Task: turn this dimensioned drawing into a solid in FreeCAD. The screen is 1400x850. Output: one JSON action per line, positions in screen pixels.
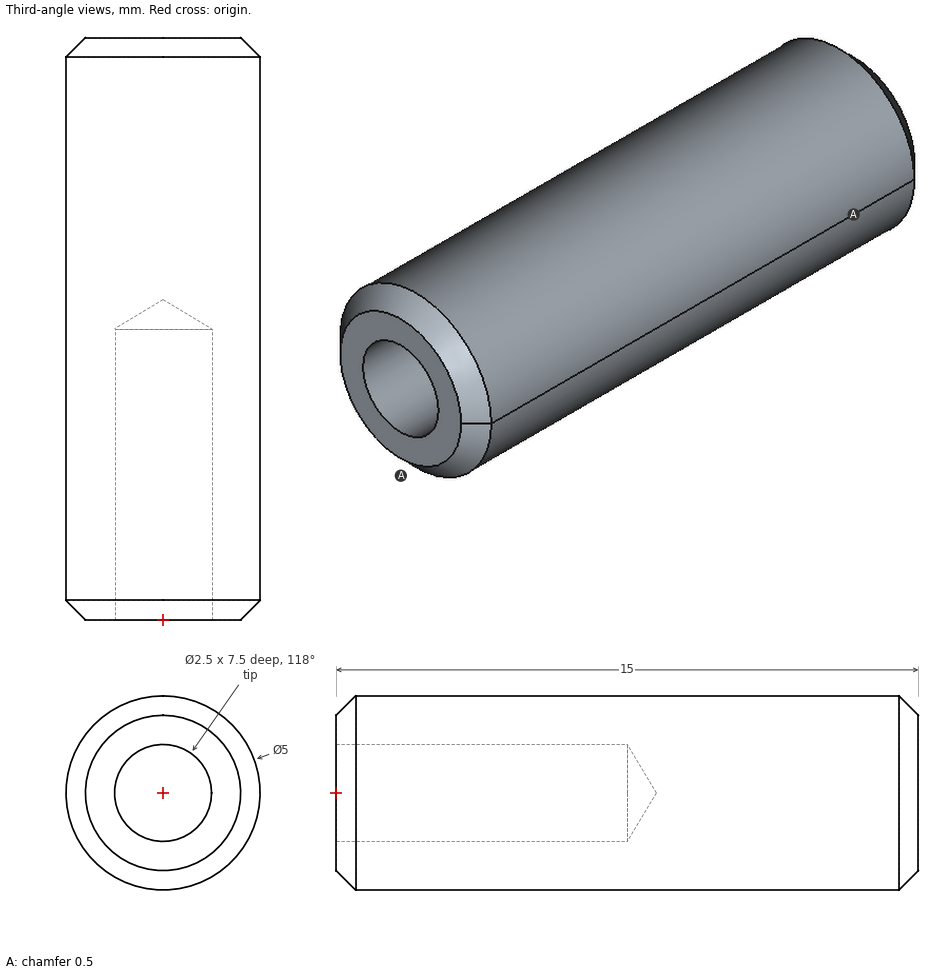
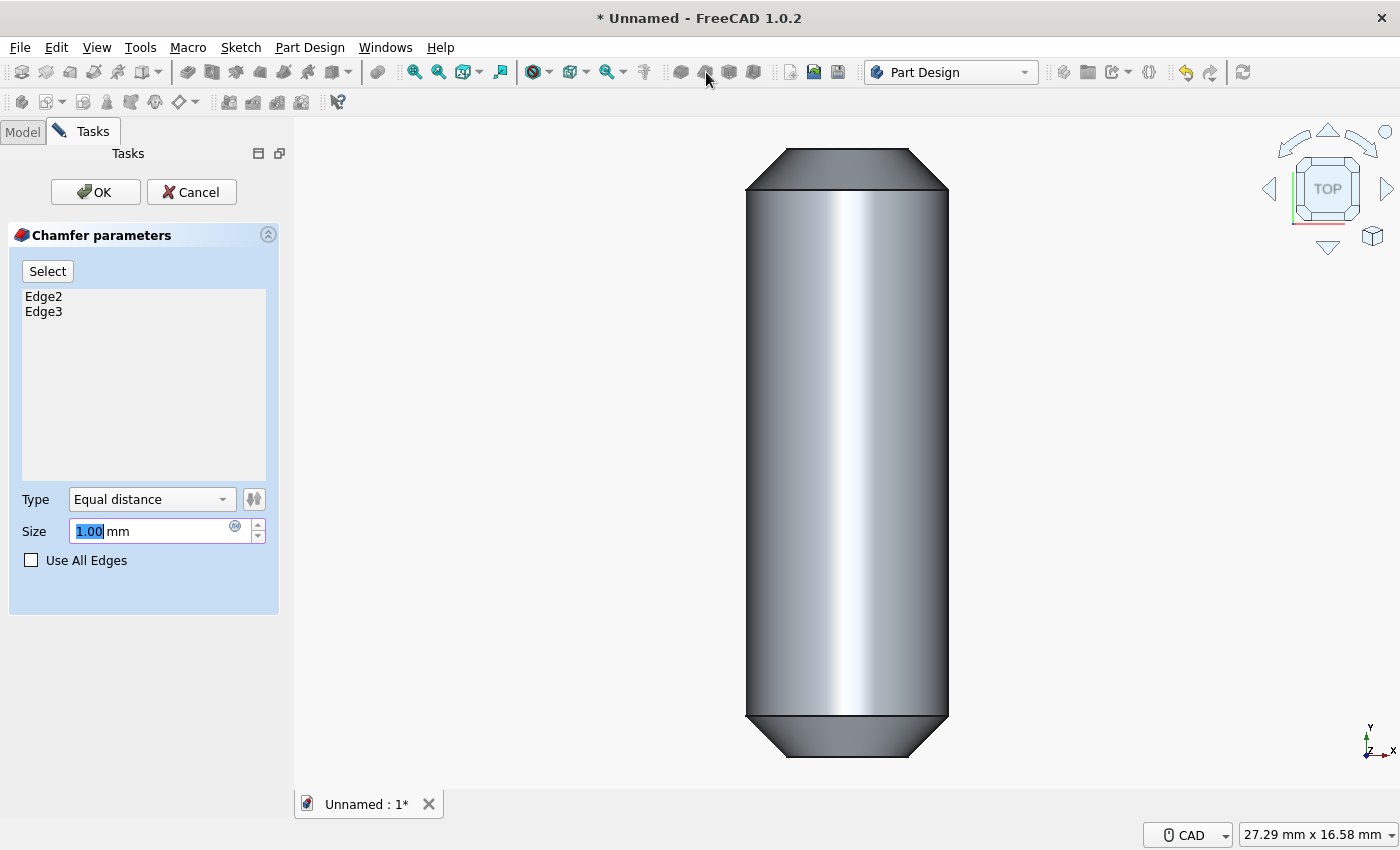
{"action": "type", "text": "0.5"}
{"action": "key", "text": "Tab"}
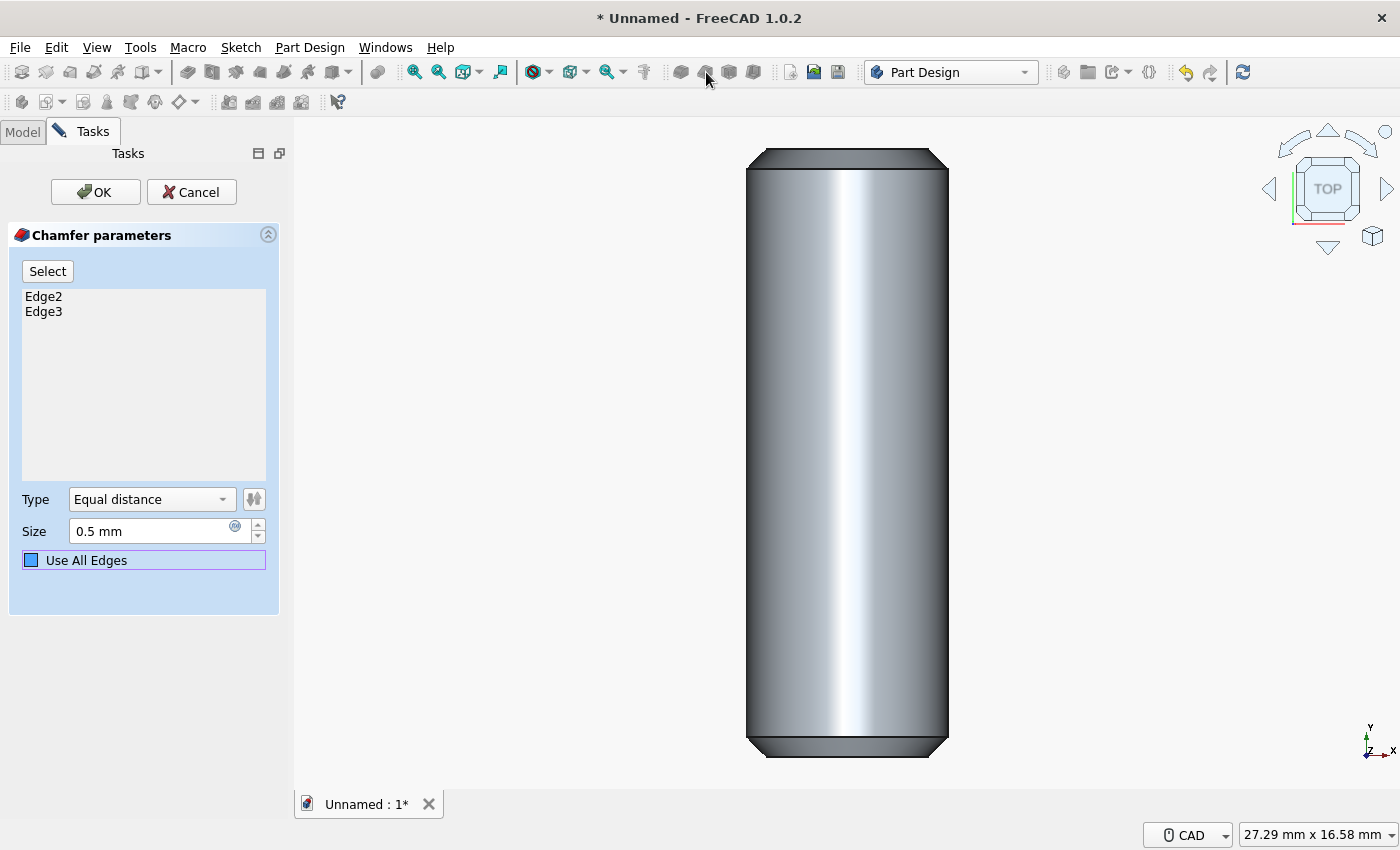
{"action": "left_click", "coordinate": [96, 192]}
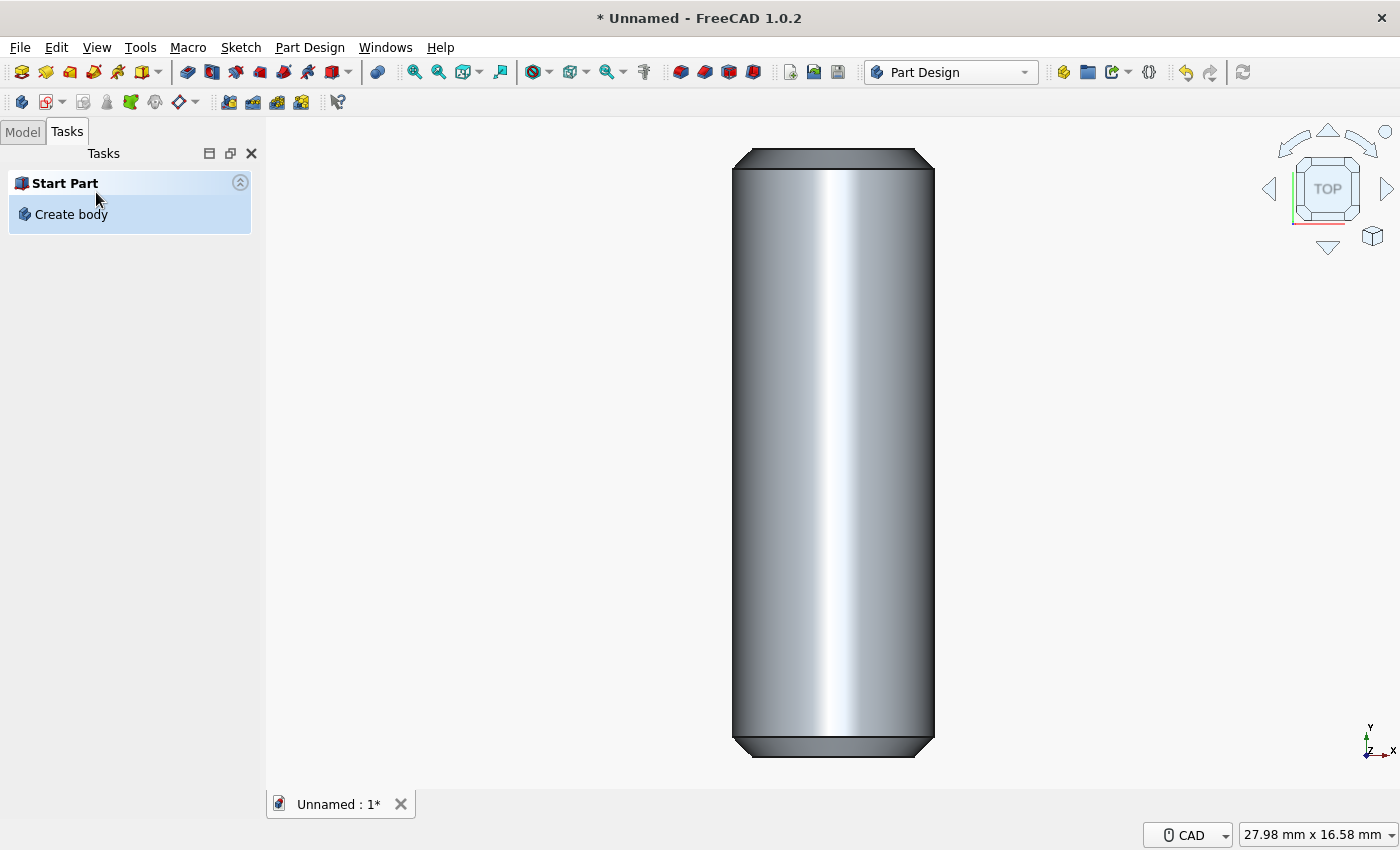
{"action": "key", "text": "0"}